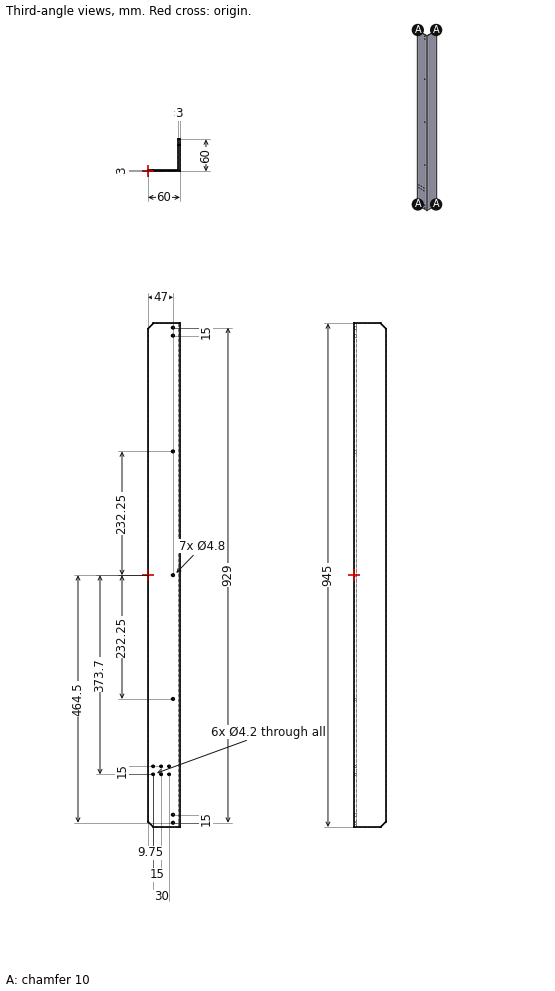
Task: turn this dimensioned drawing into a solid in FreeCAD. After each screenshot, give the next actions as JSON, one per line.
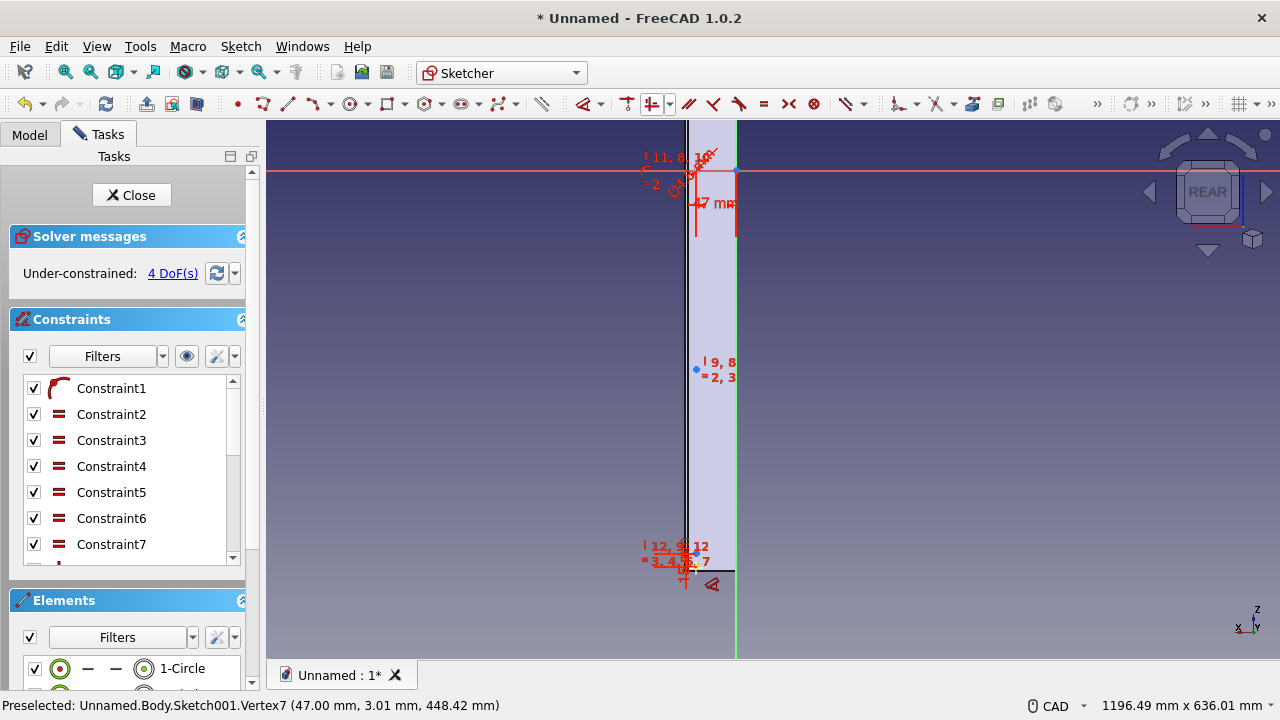
{"action": "left_click", "coordinate": [696, 567]}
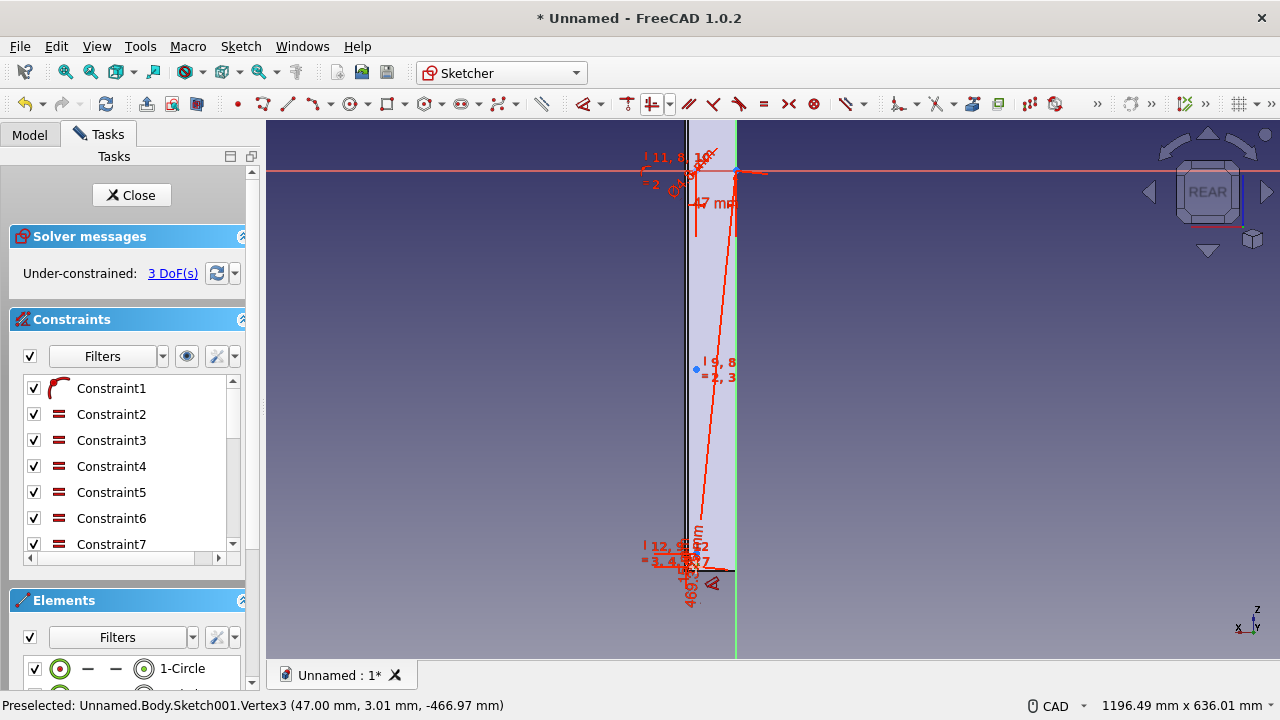
{"action": "scroll", "coordinate": [696, 568], "scroll_direction": "down", "scroll_amount": 4}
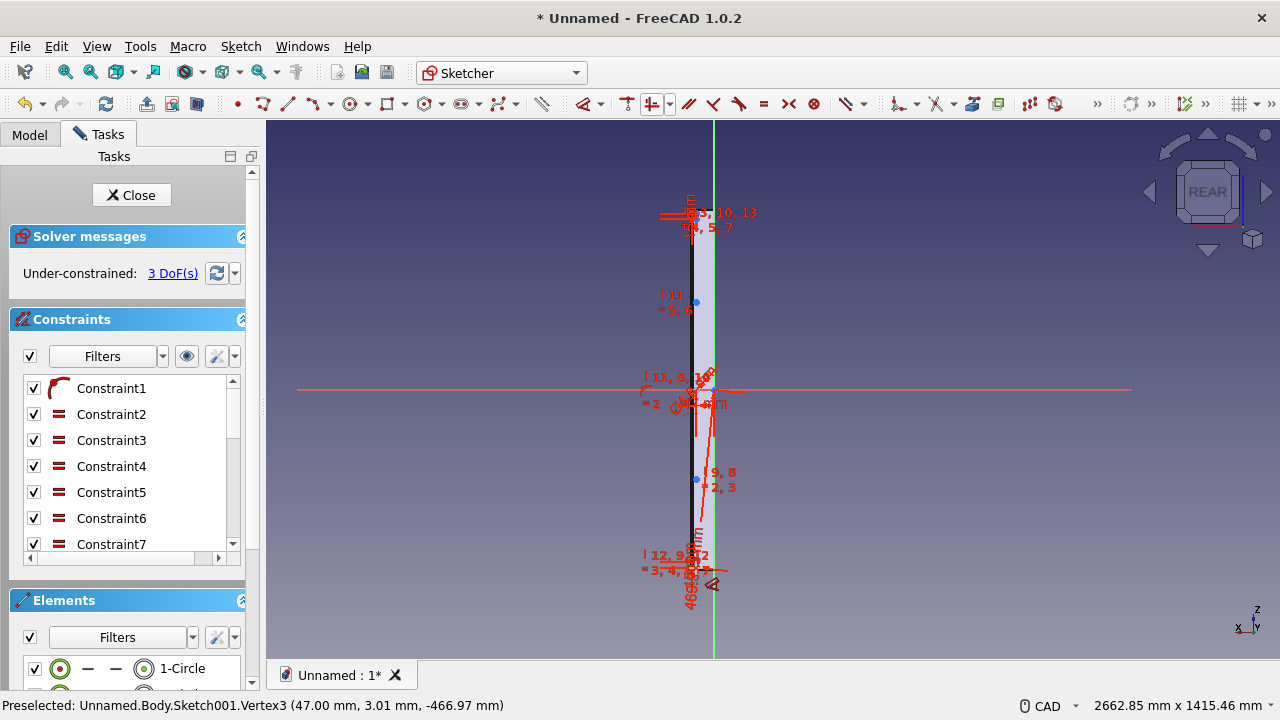
{"action": "scroll", "coordinate": [696, 214], "scroll_direction": "up", "scroll_amount": 4}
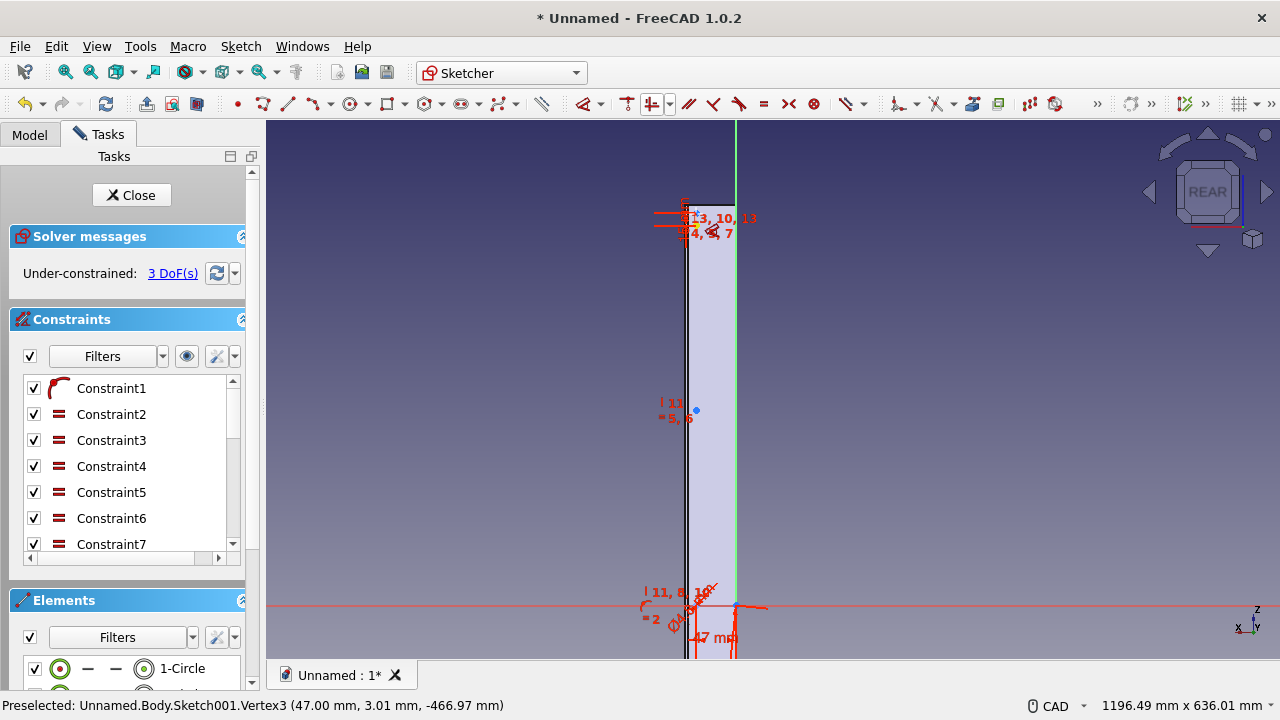
{"action": "left_click", "coordinate": [696, 213]}
{"action": "left_click", "coordinate": [662, 422]}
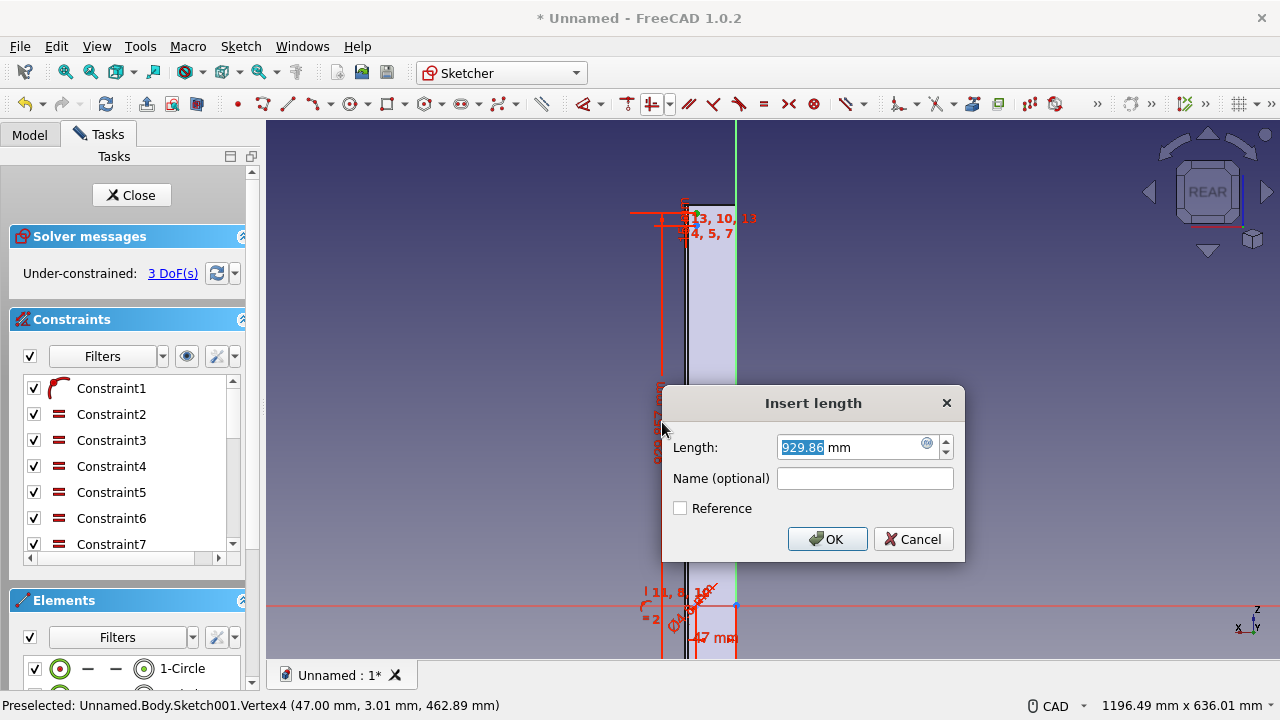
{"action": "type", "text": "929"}
{"action": "key", "text": "Return"}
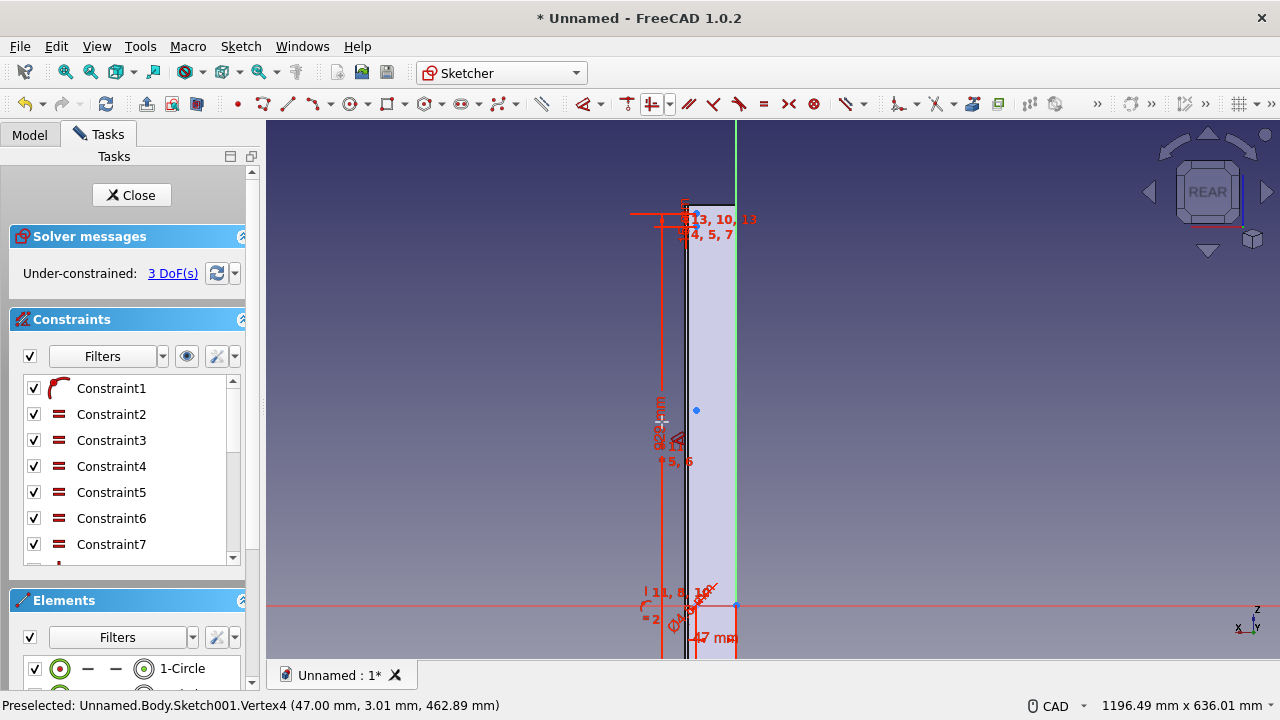
{"action": "scroll", "coordinate": [696, 213], "scroll_direction": "down", "scroll_amount": 4}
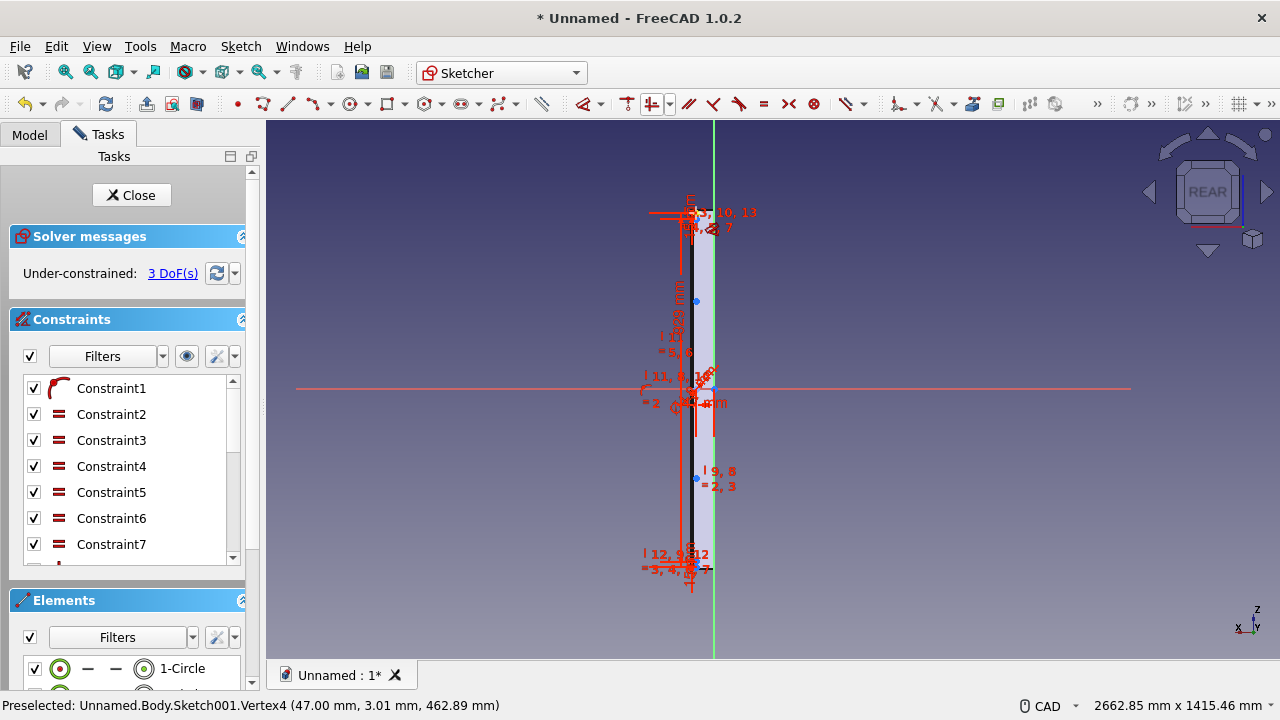
{"action": "scroll", "coordinate": [696, 567], "scroll_direction": "up", "scroll_amount": 4}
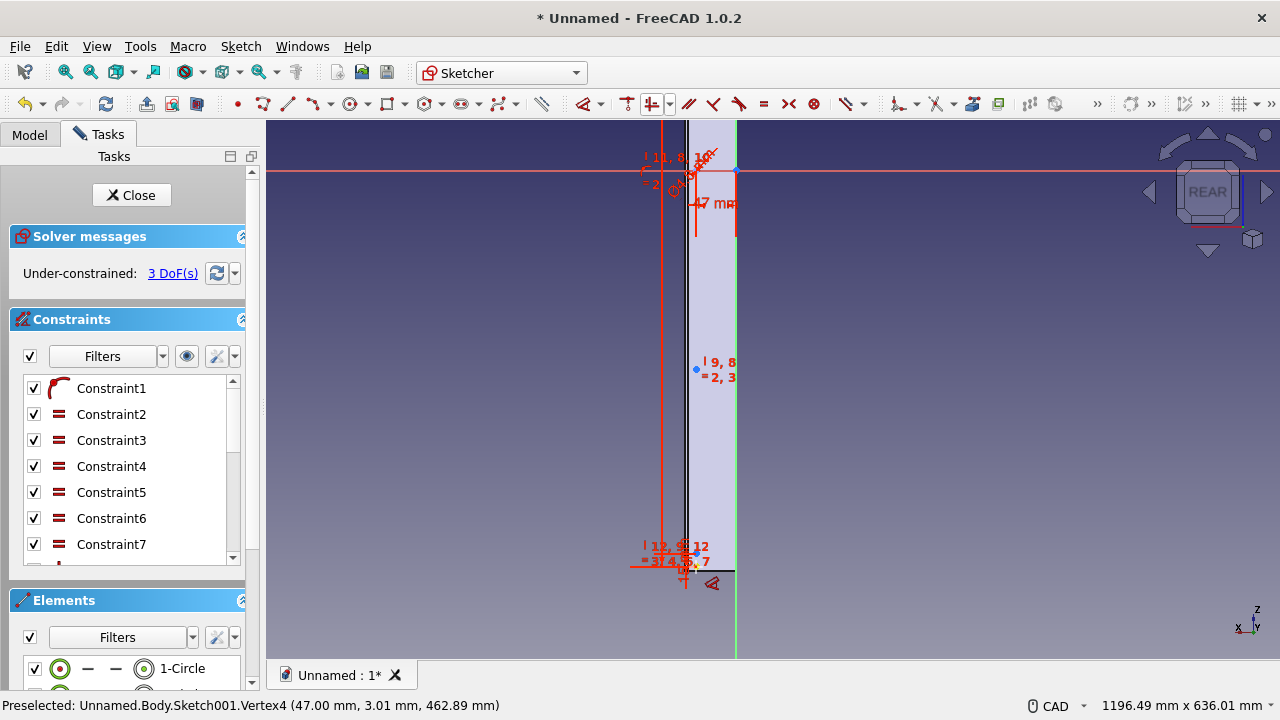
{"action": "left_click", "coordinate": [696, 567]}
{"action": "left_click", "coordinate": [770, 369]}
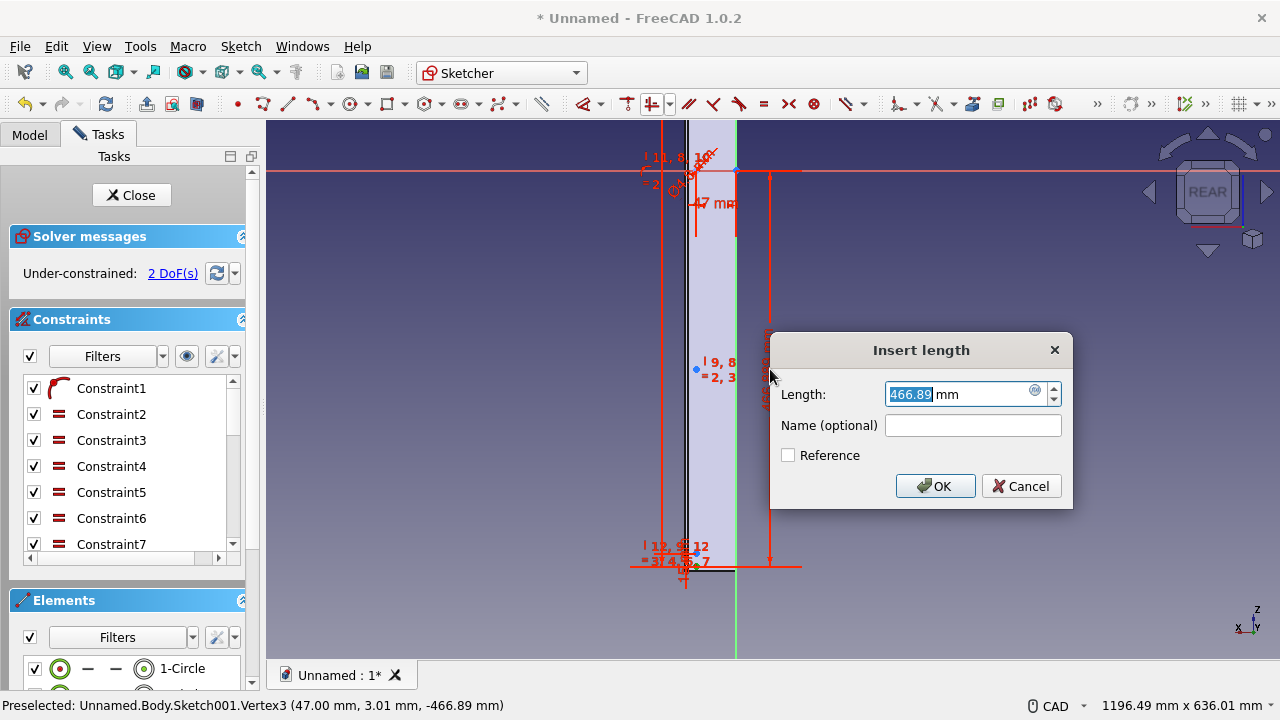
{"action": "type", "text": "464.5"}
{"action": "key", "text": "Return"}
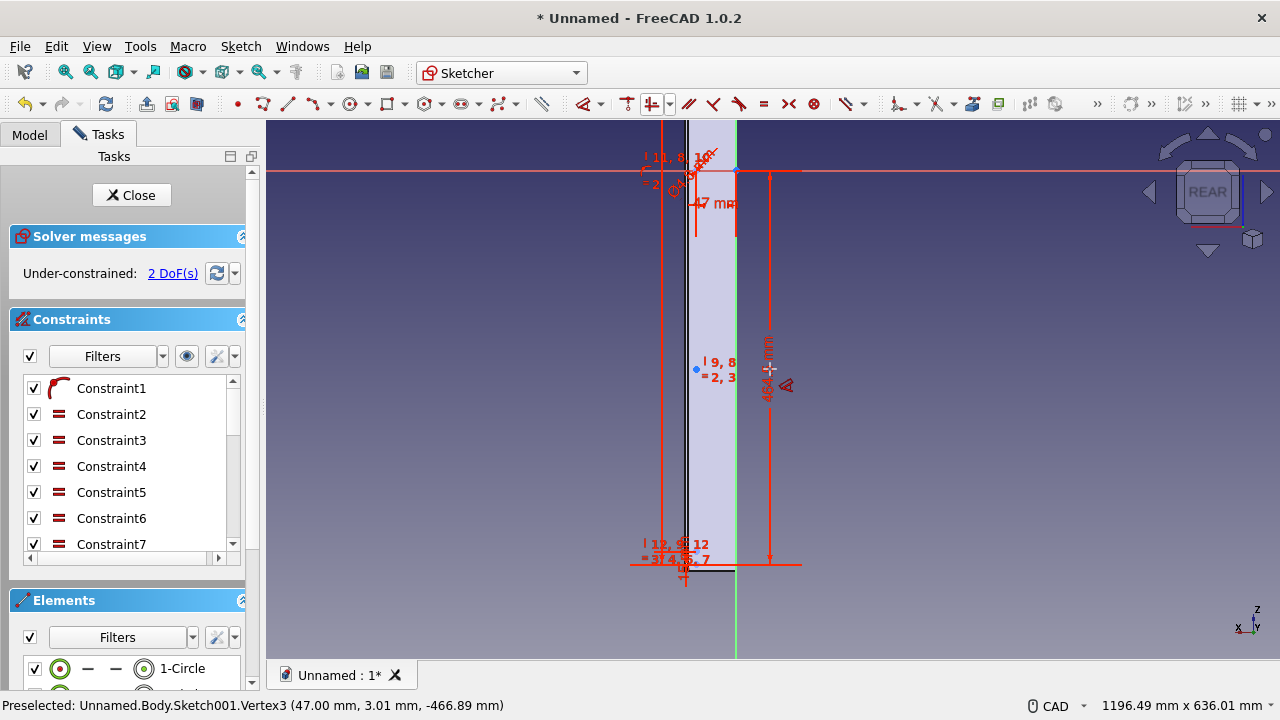
{"action": "left_click", "coordinate": [696, 369]}
{"action": "left_click", "coordinate": [770, 270]}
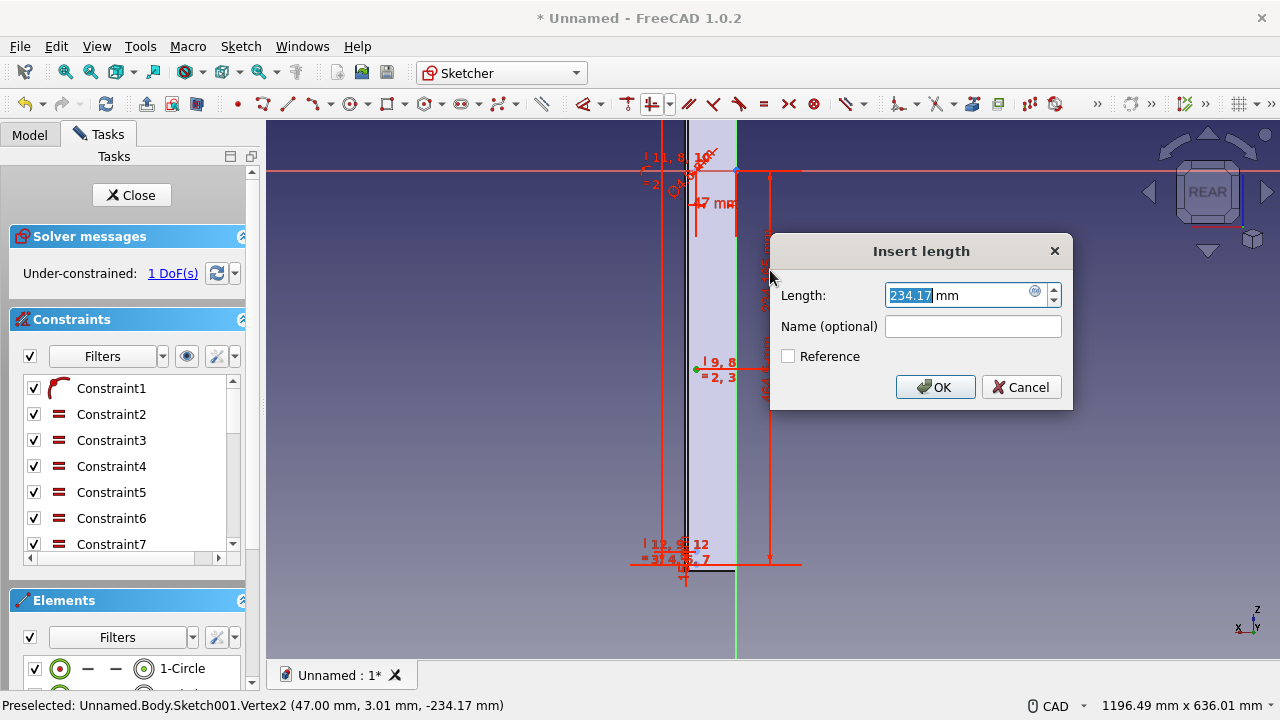
{"action": "type", "text": "232.25"}
{"action": "key", "text": "Return"}